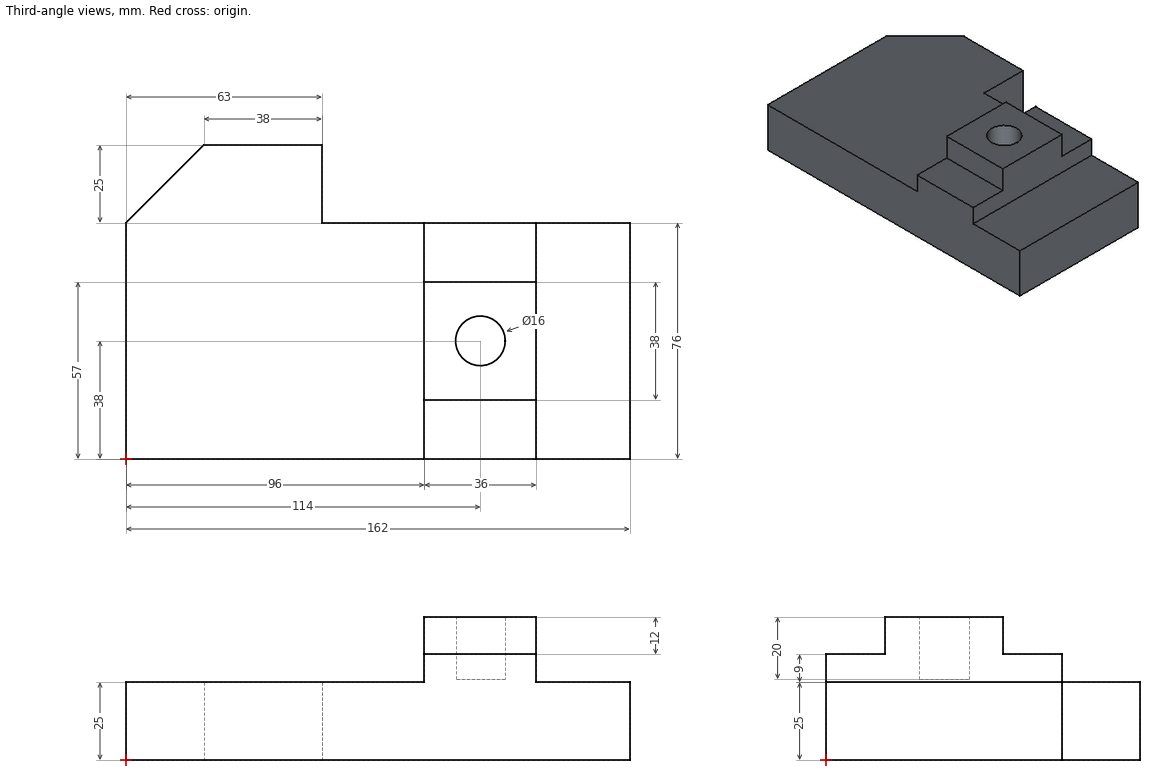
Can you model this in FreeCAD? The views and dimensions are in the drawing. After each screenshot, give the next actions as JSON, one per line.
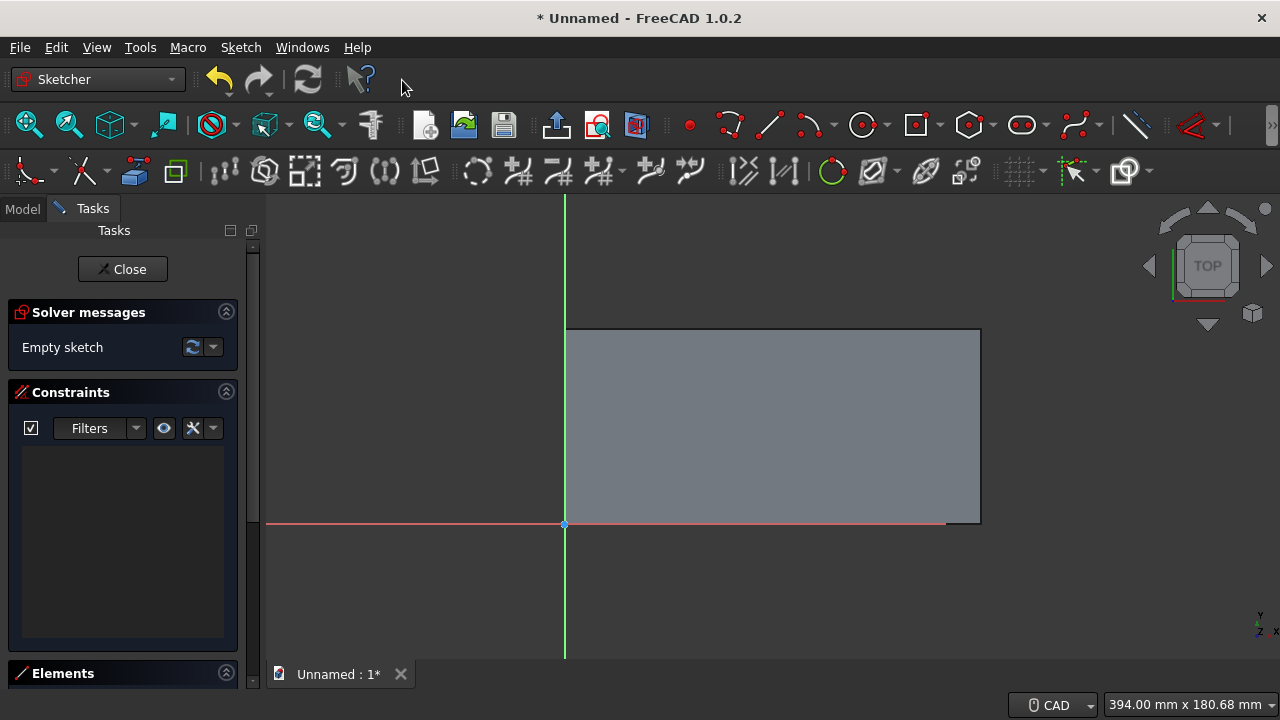
{"action": "left_click", "coordinate": [565, 329]}
{"action": "left_click", "coordinate": [727, 329]}
{"action": "left_click", "coordinate": [727, 264]}
{"action": "left_click", "coordinate": [629, 264]}
{"action": "left_click", "coordinate": [565, 330]}
{"action": "key", "text": "Escape"}
{"action": "key", "text": "Escape"}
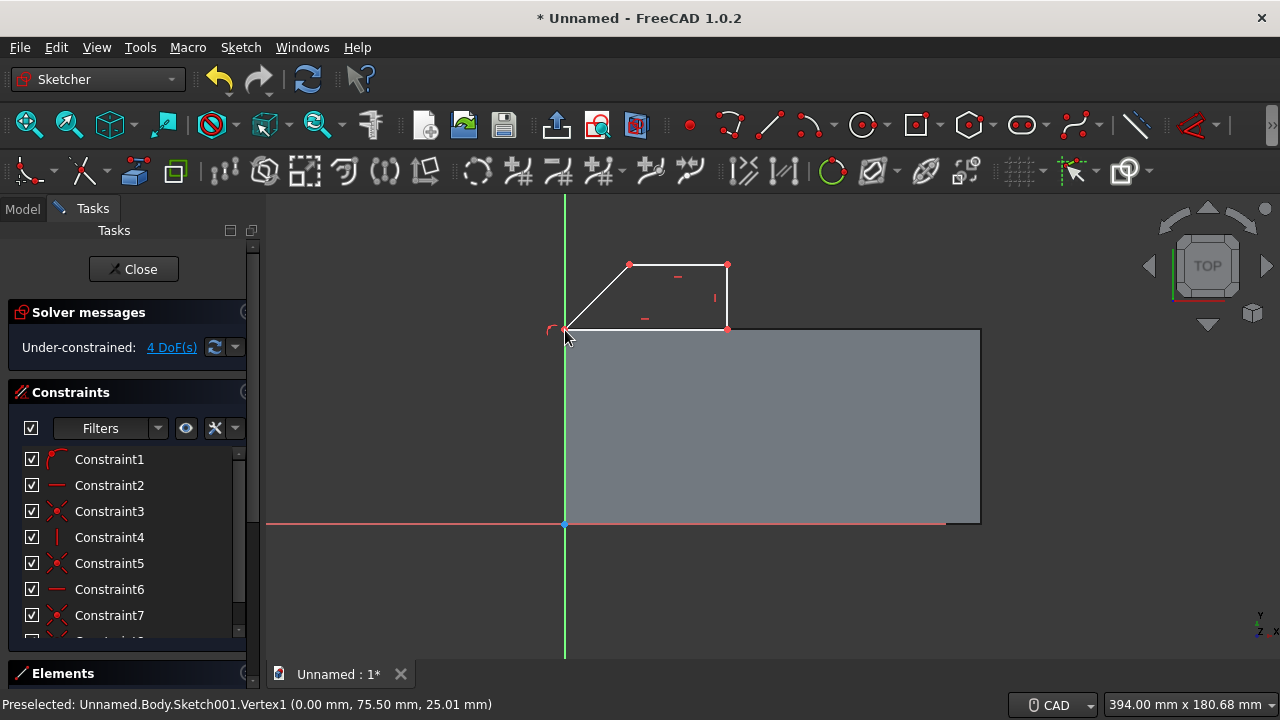
{"action": "left_click", "coordinate": [613, 330]}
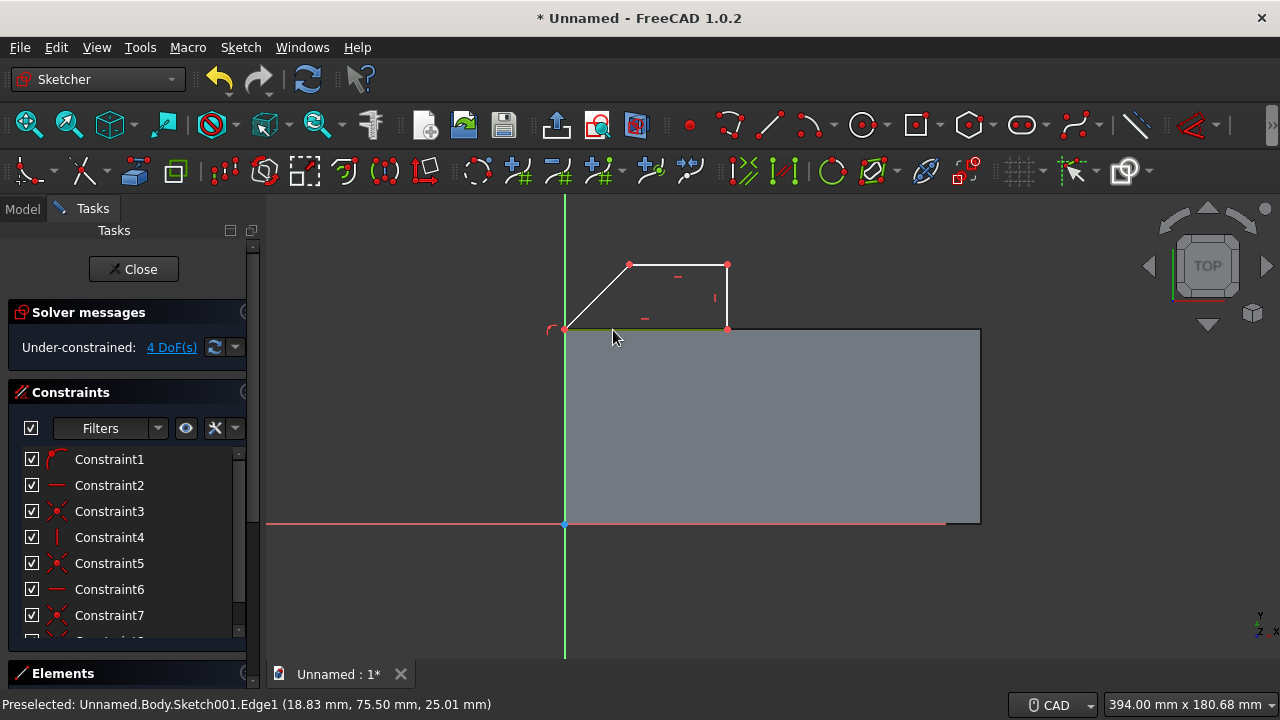
{"action": "key", "text": "l"}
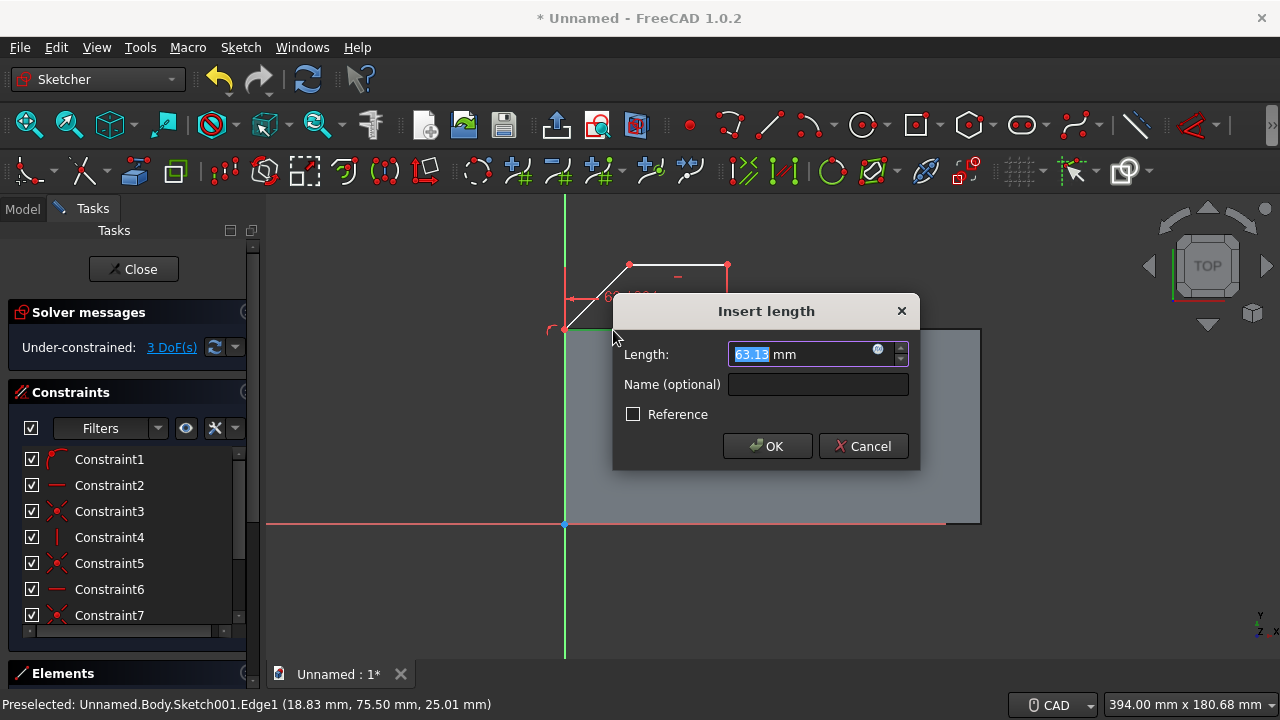
{"action": "type", "text": "63"}
{"action": "key", "text": "Return"}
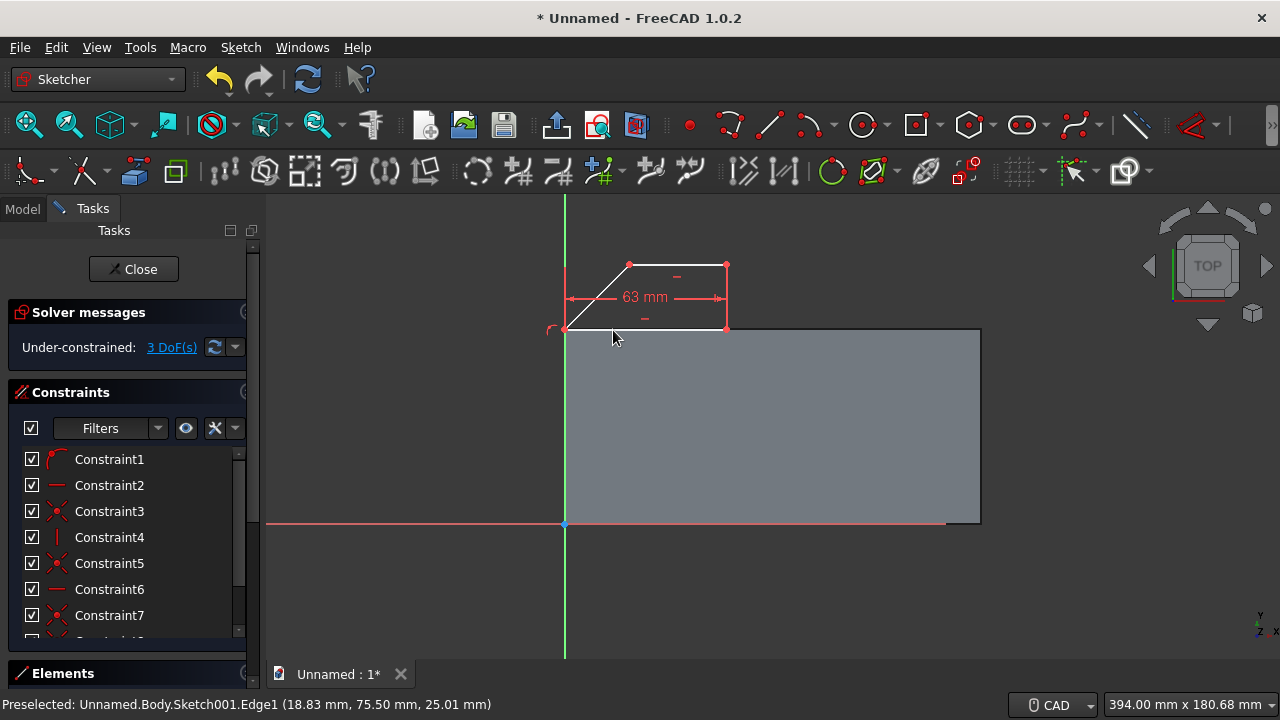
{"action": "left_click", "coordinate": [727, 311]}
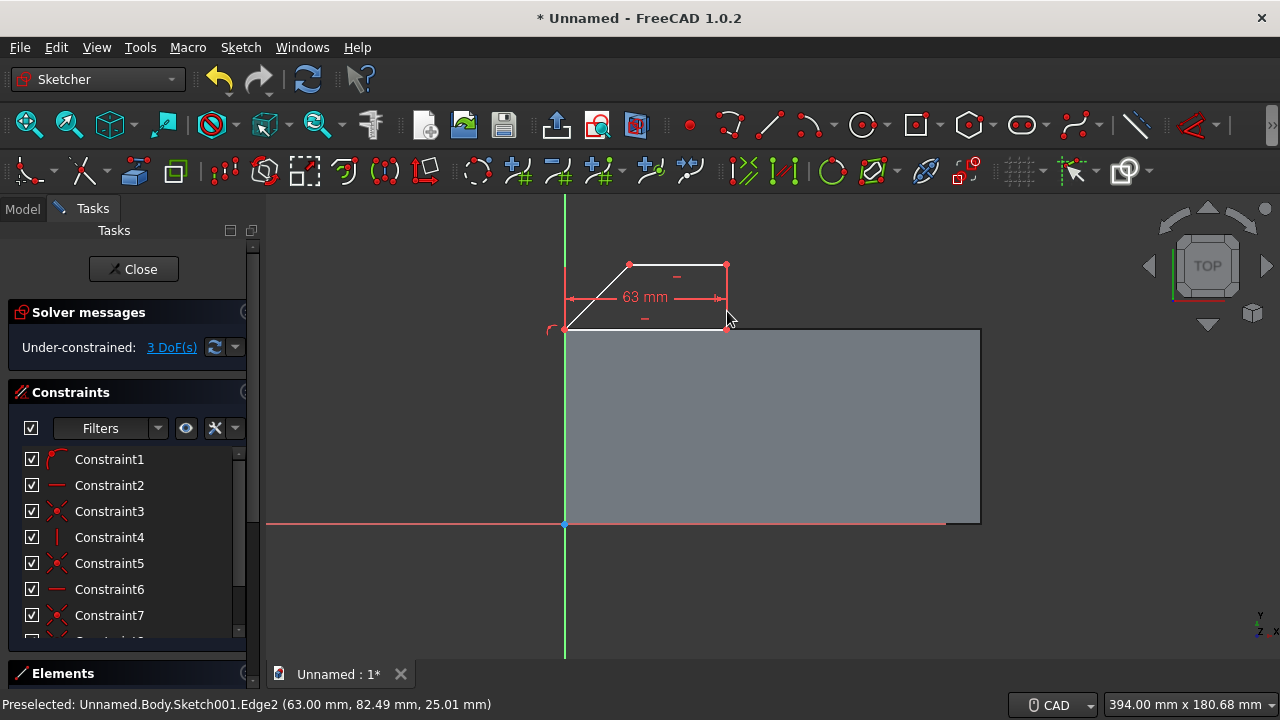
{"action": "key", "text": "i"}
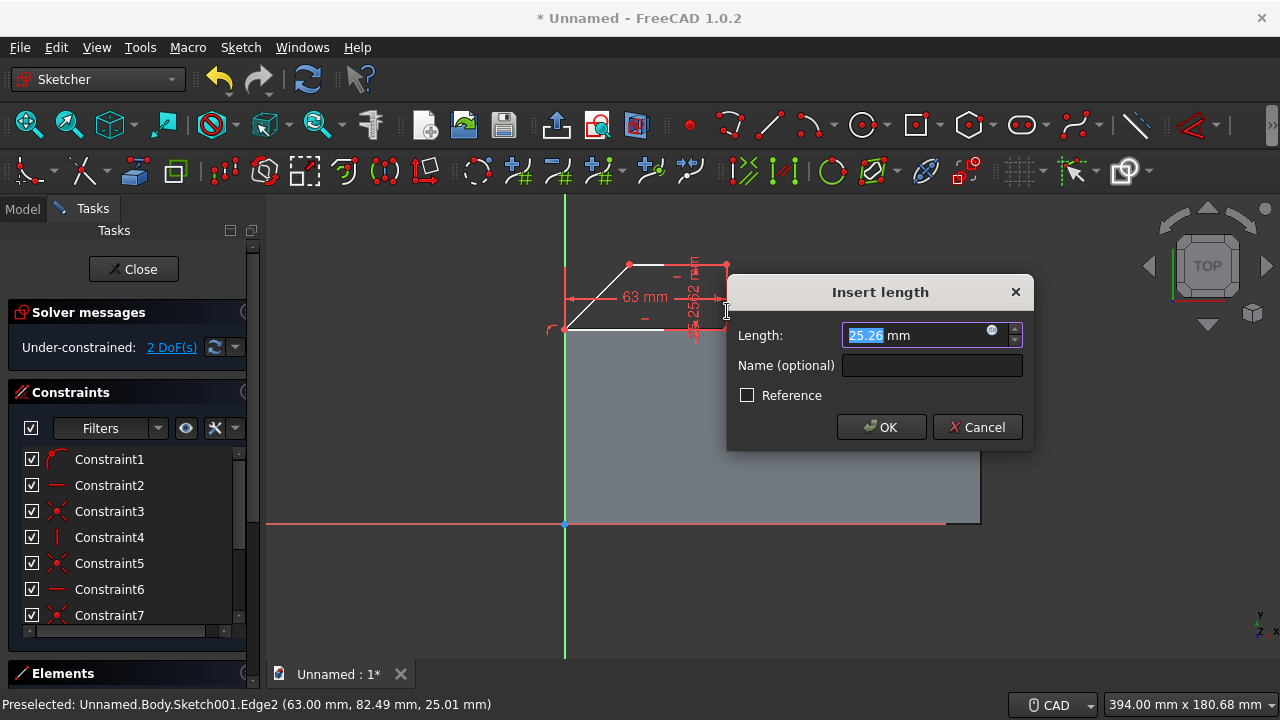
{"action": "type", "text": "25"}
{"action": "key", "text": "Return"}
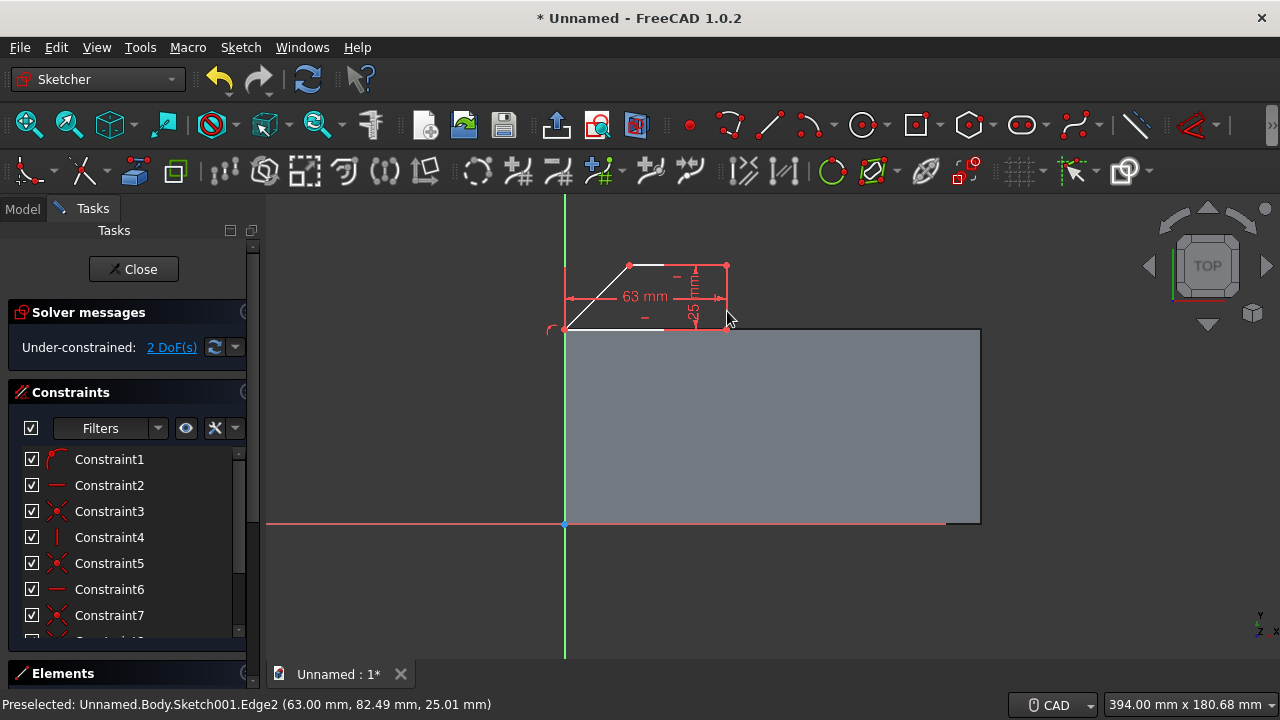
{"action": "left_click", "coordinate": [697, 265]}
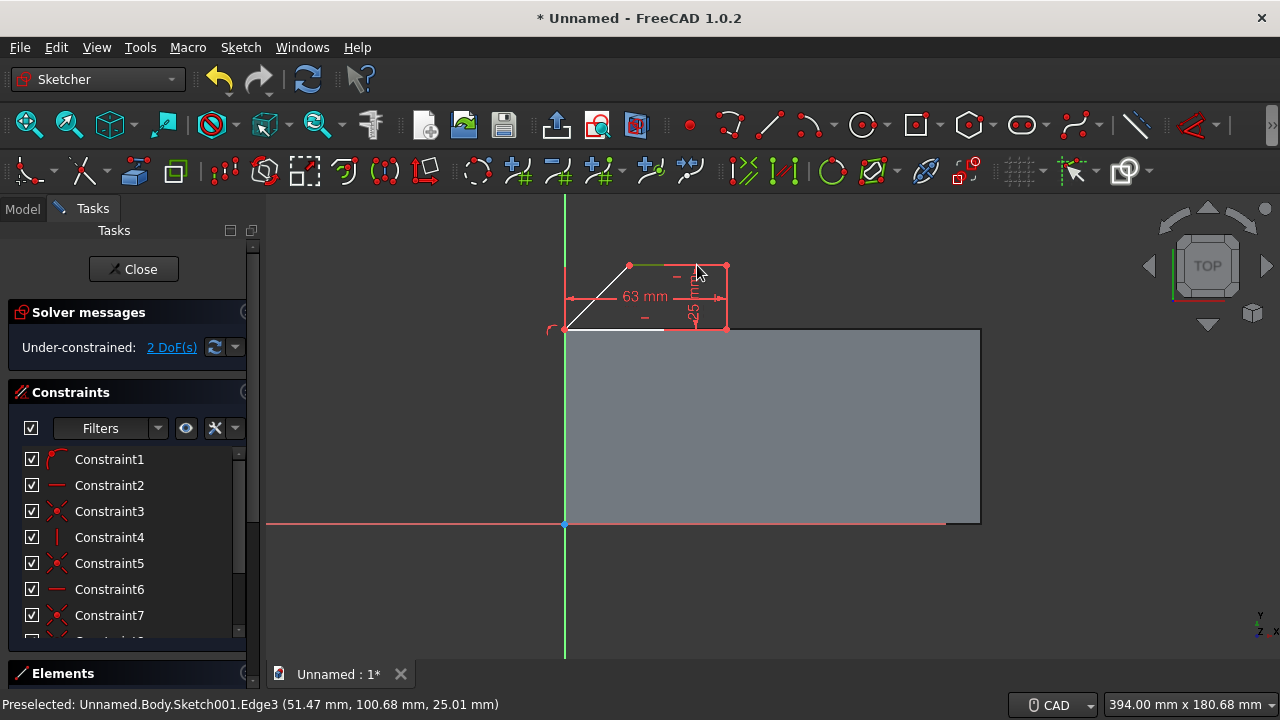
{"action": "key", "text": "l"}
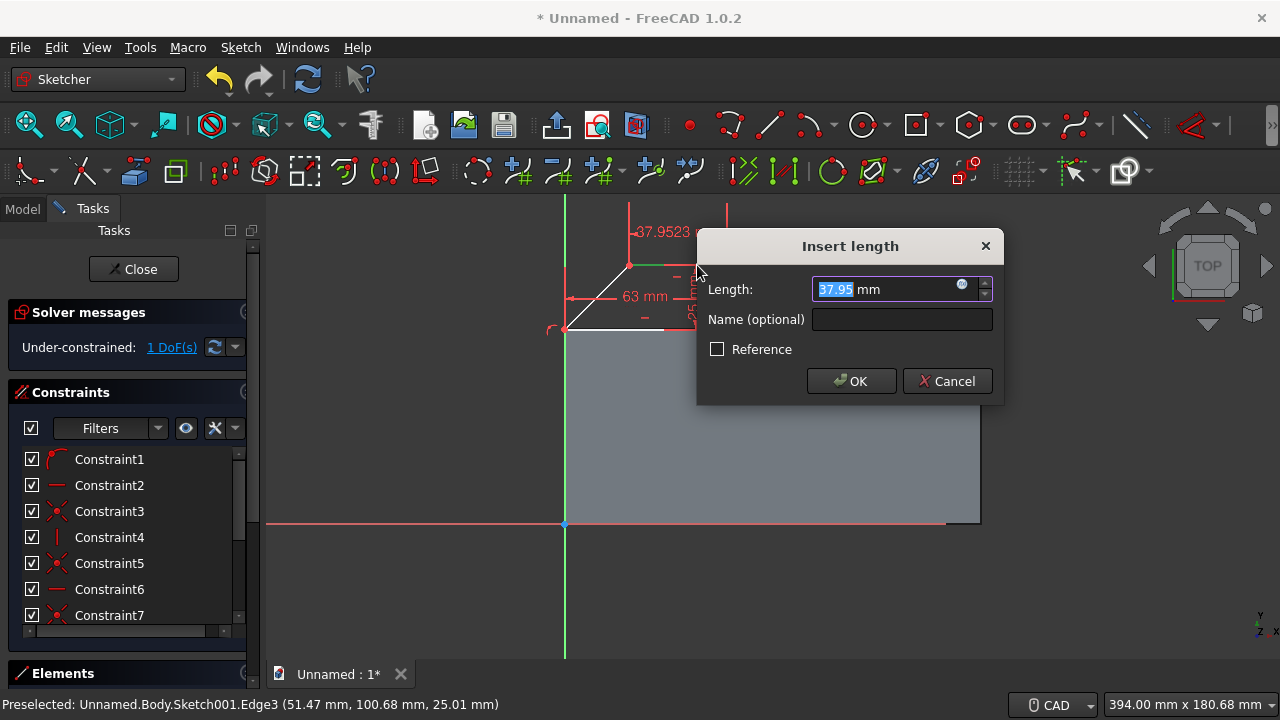
{"action": "type", "text": "38"}
{"action": "key", "text": "Return"}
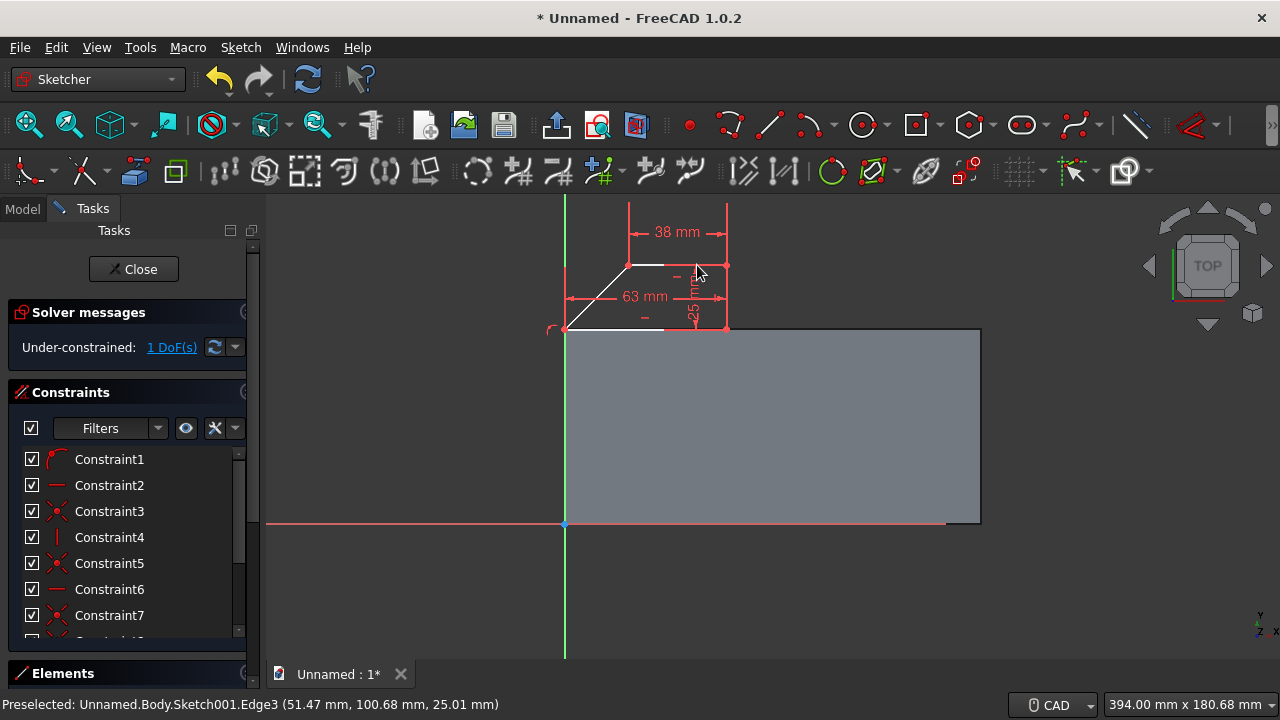
{"action": "left_click", "coordinate": [565, 330]}